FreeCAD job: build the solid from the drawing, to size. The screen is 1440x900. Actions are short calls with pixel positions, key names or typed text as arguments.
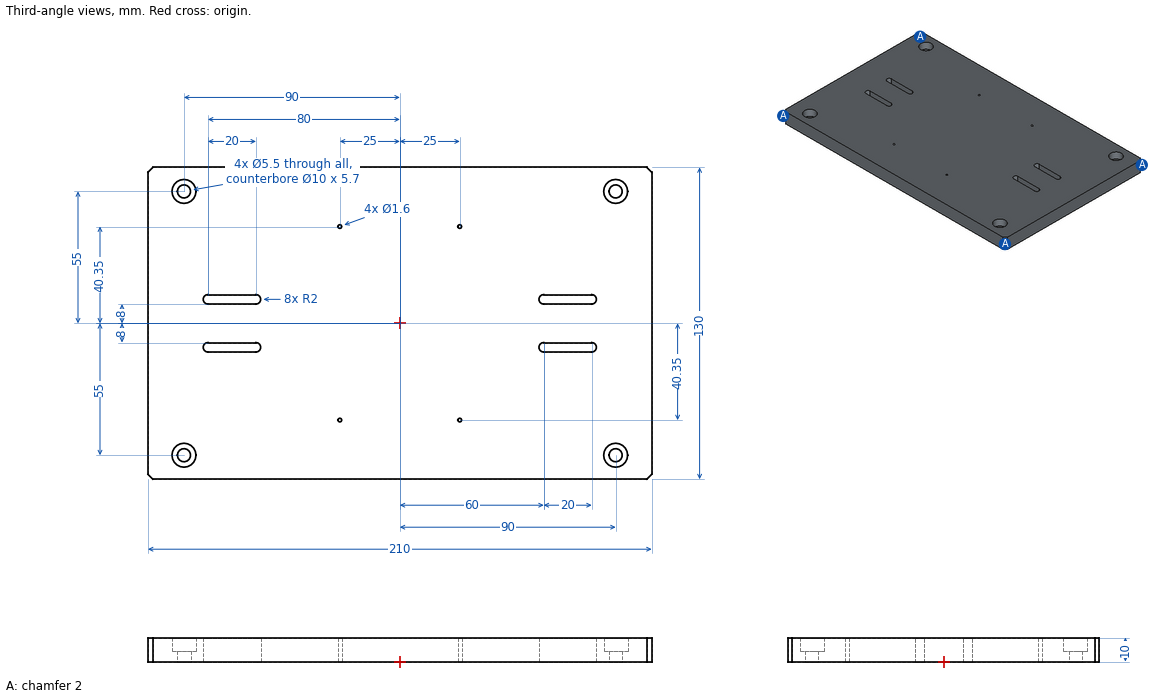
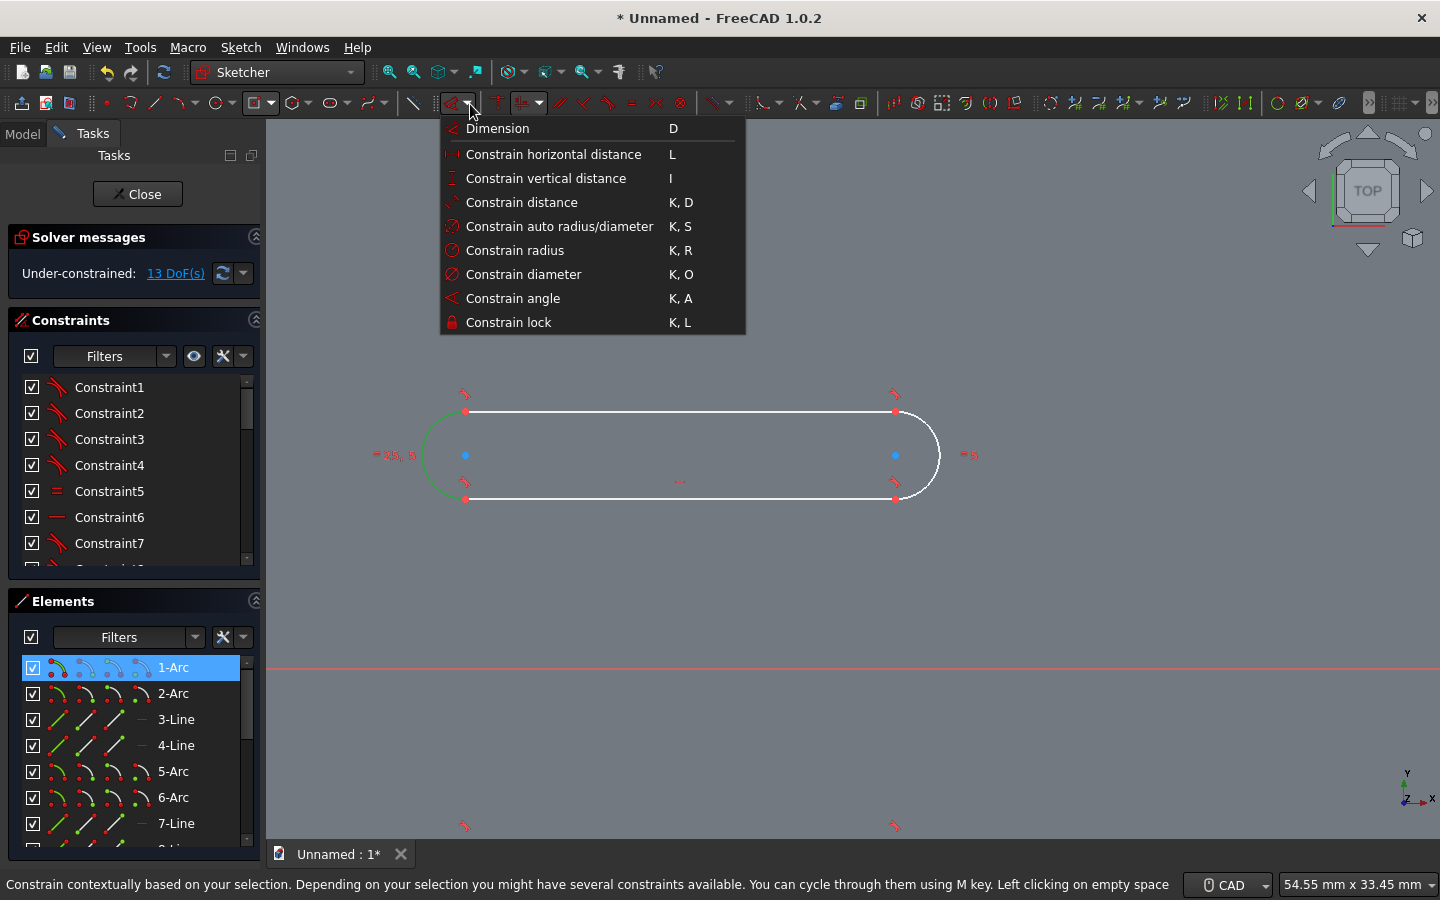
click(593, 250)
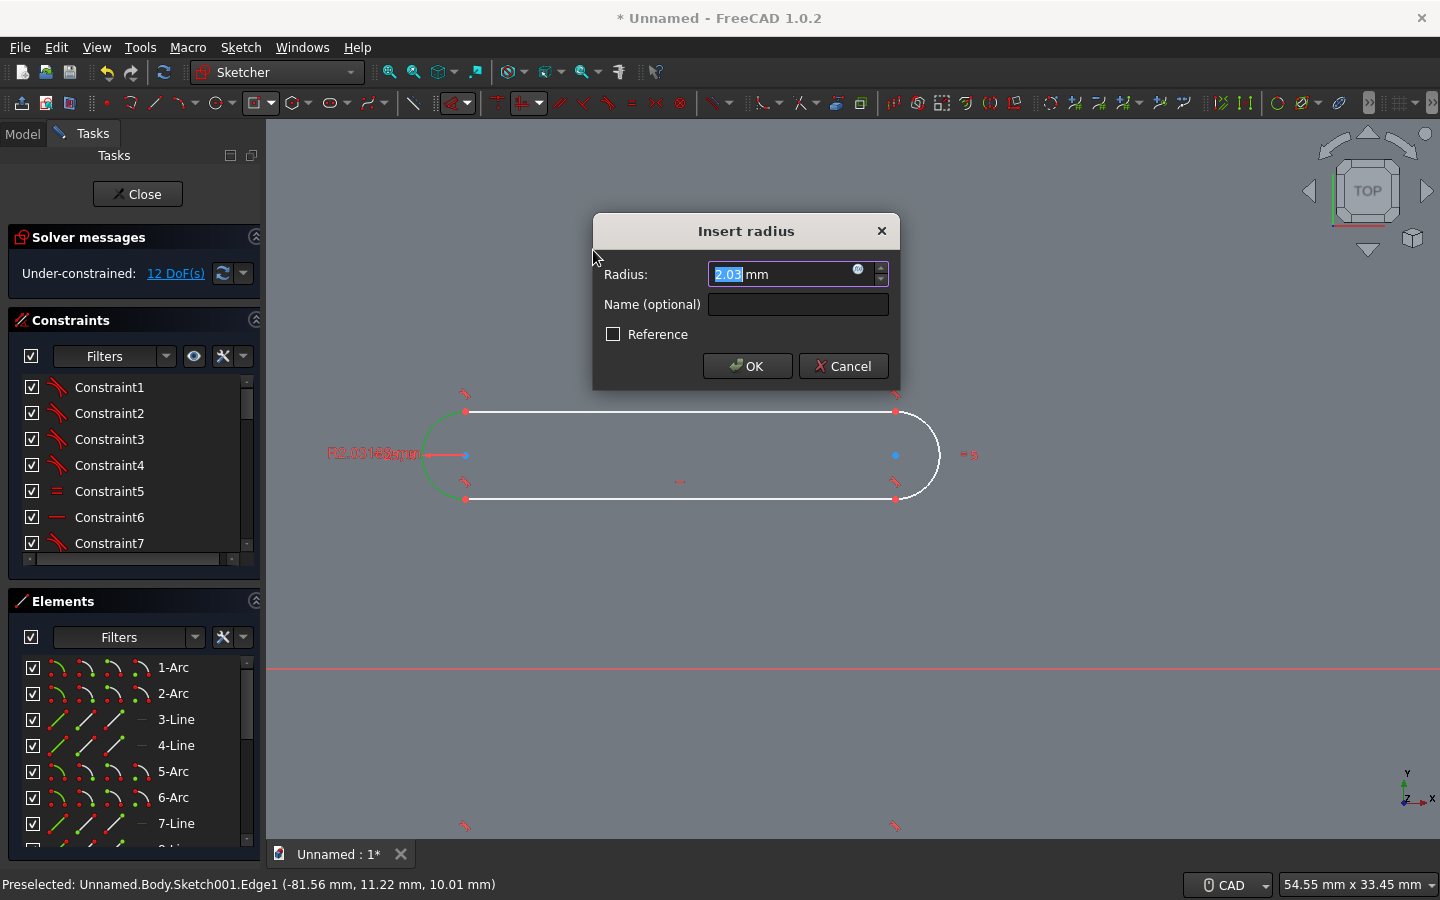
text(2)
key(Return)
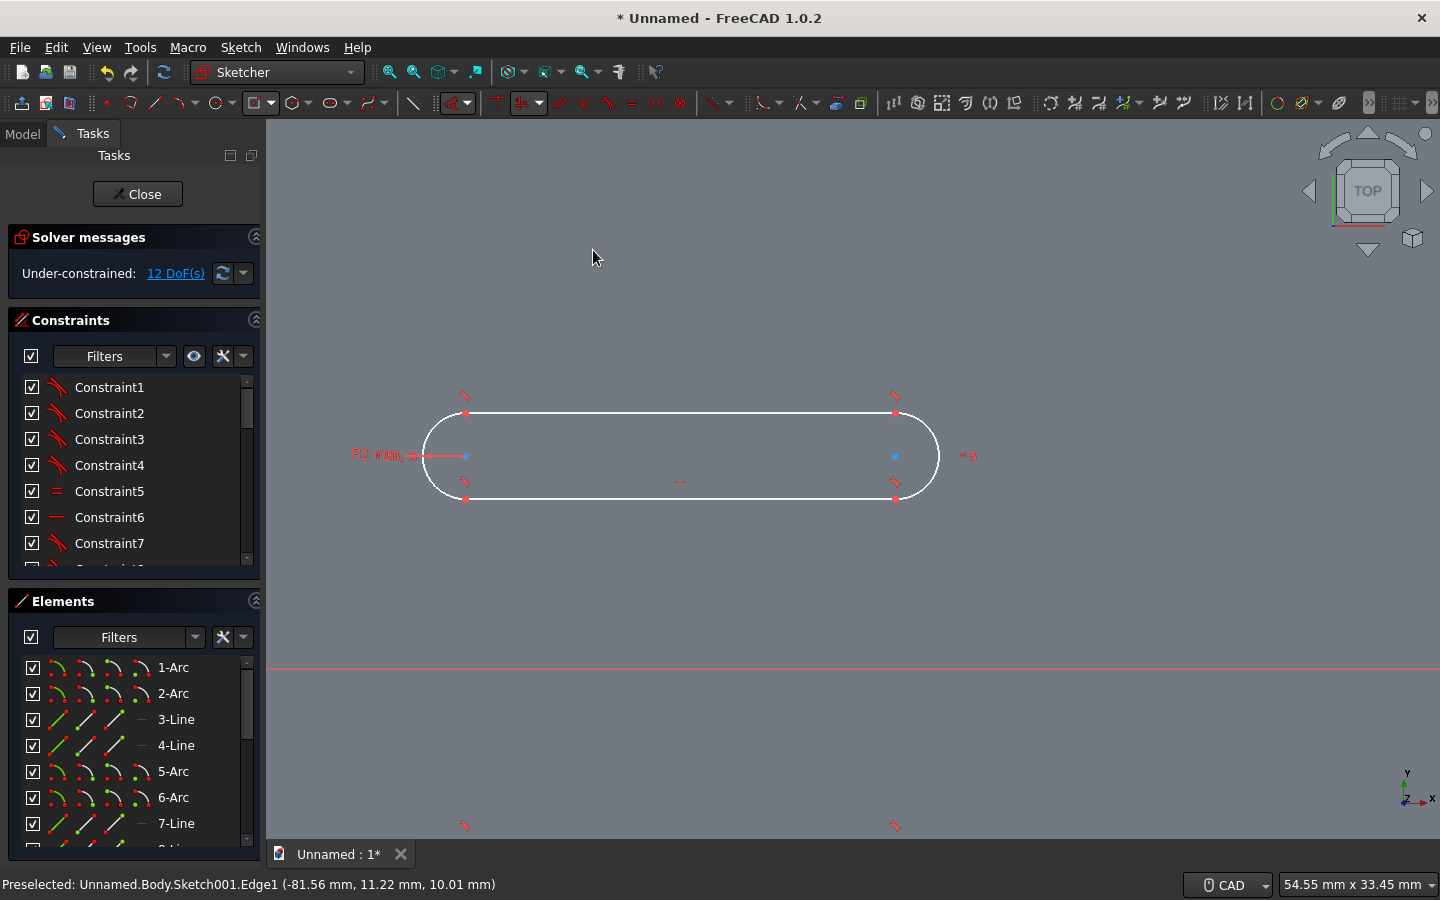
scroll(430, 431, down, 8)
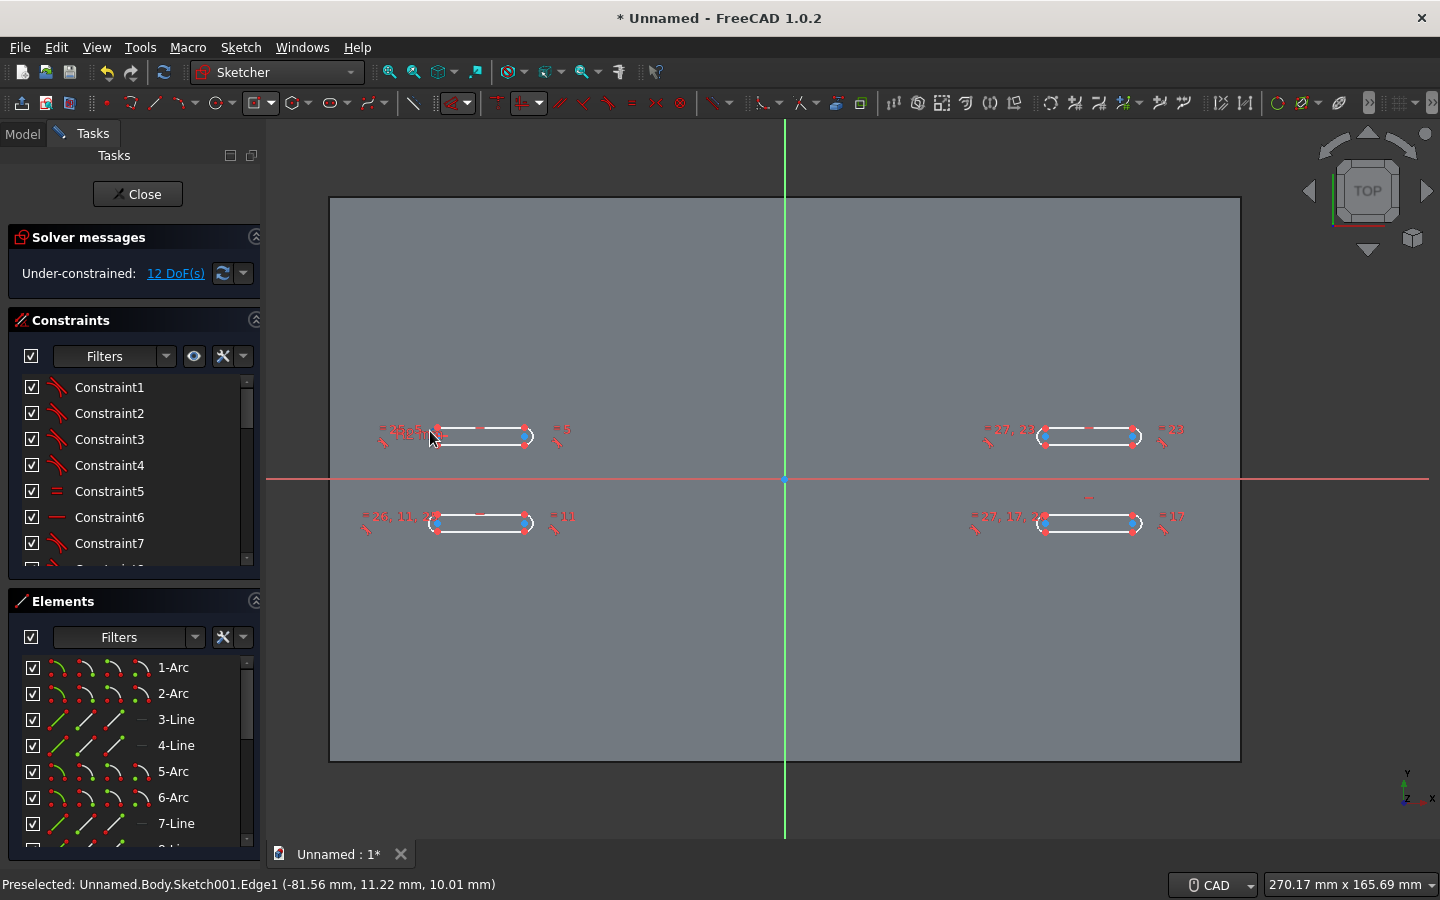
click(463, 428)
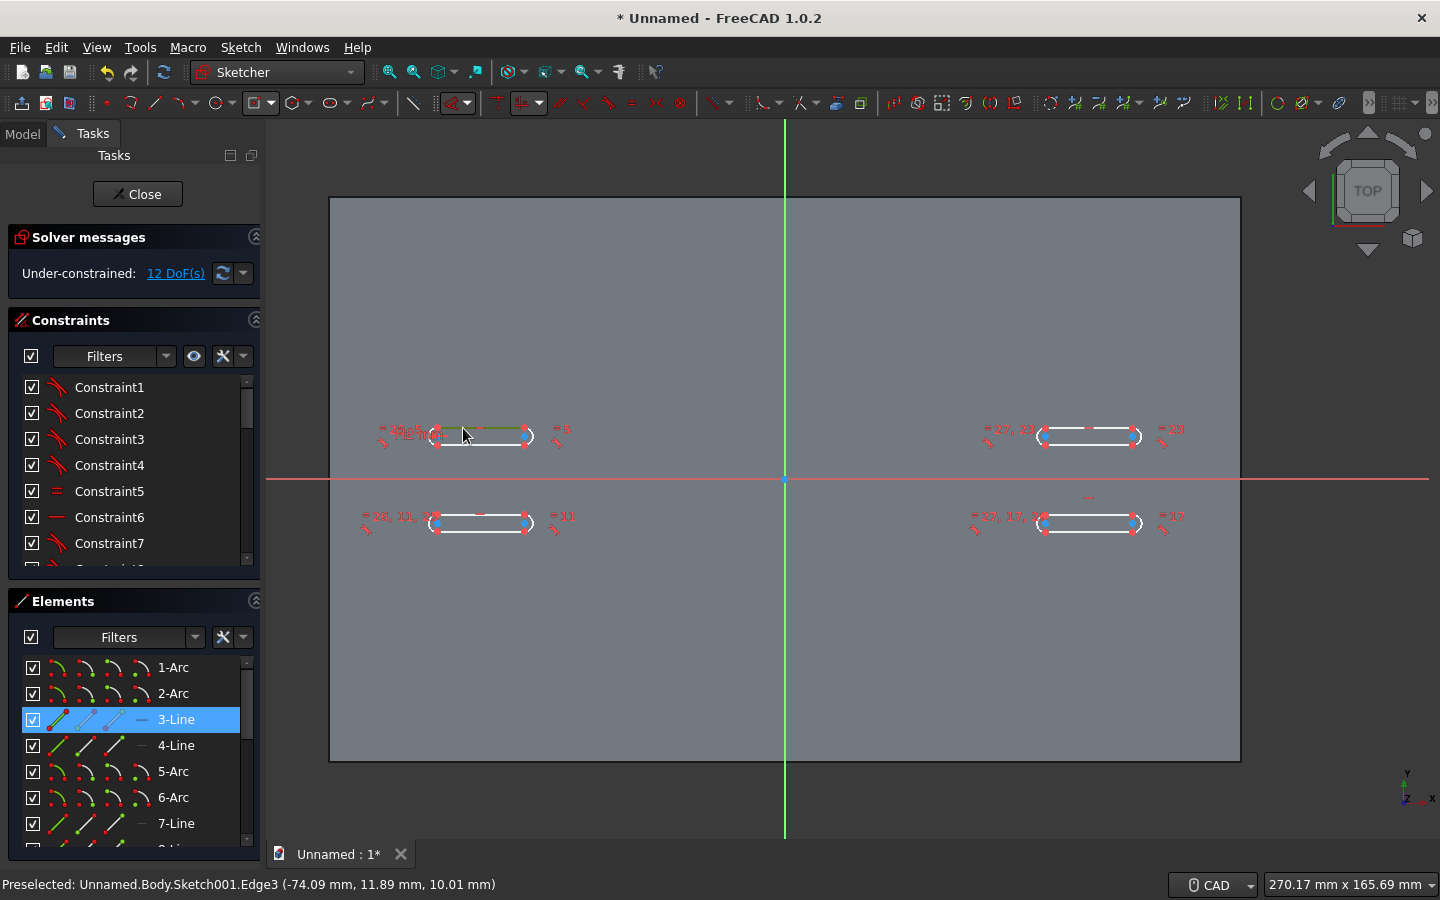
click(470, 104)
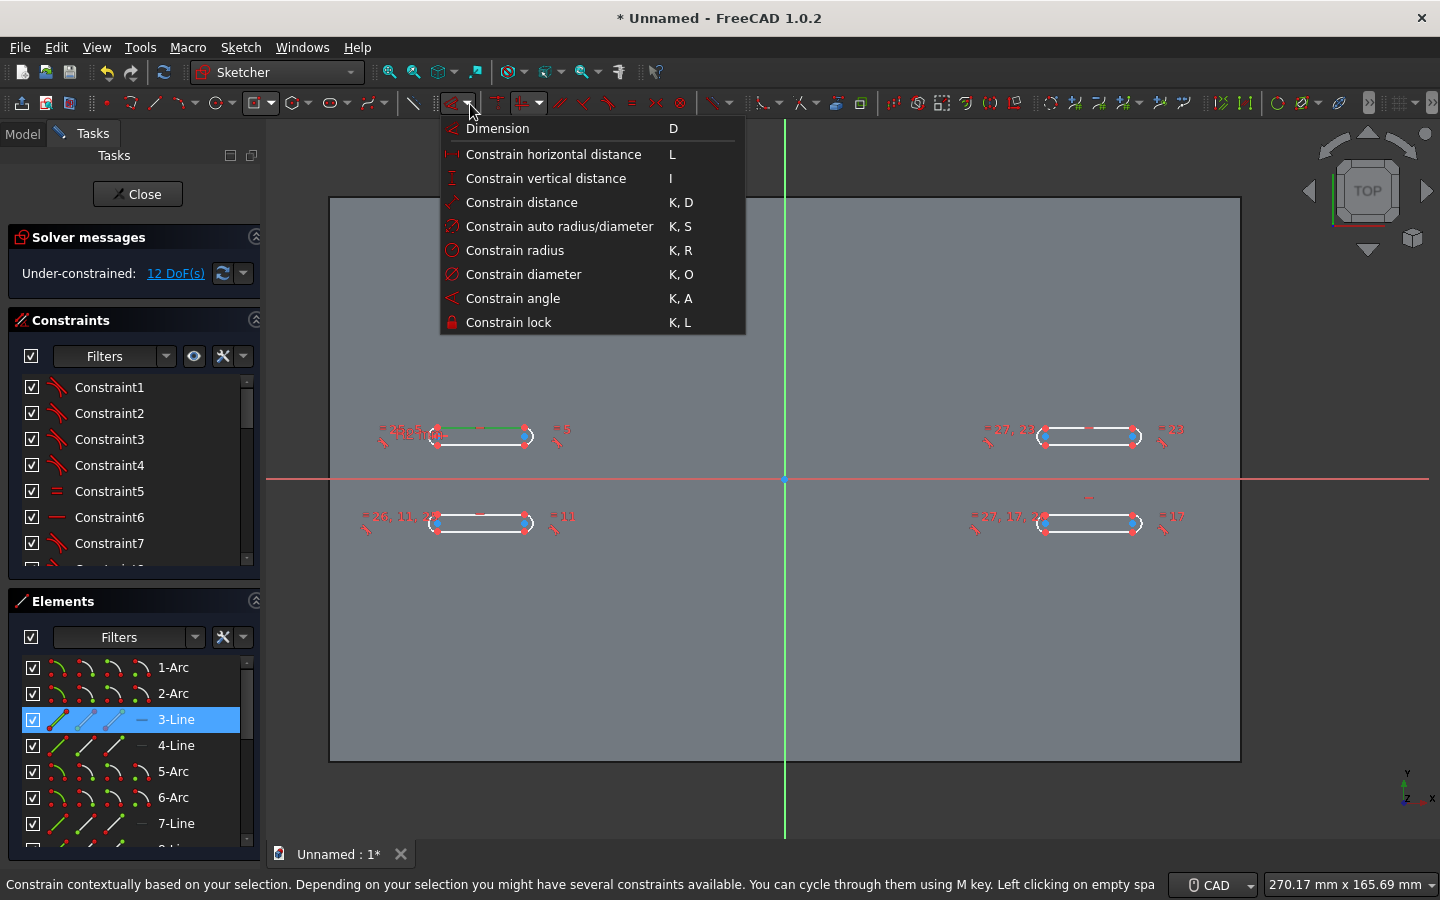
click(593, 154)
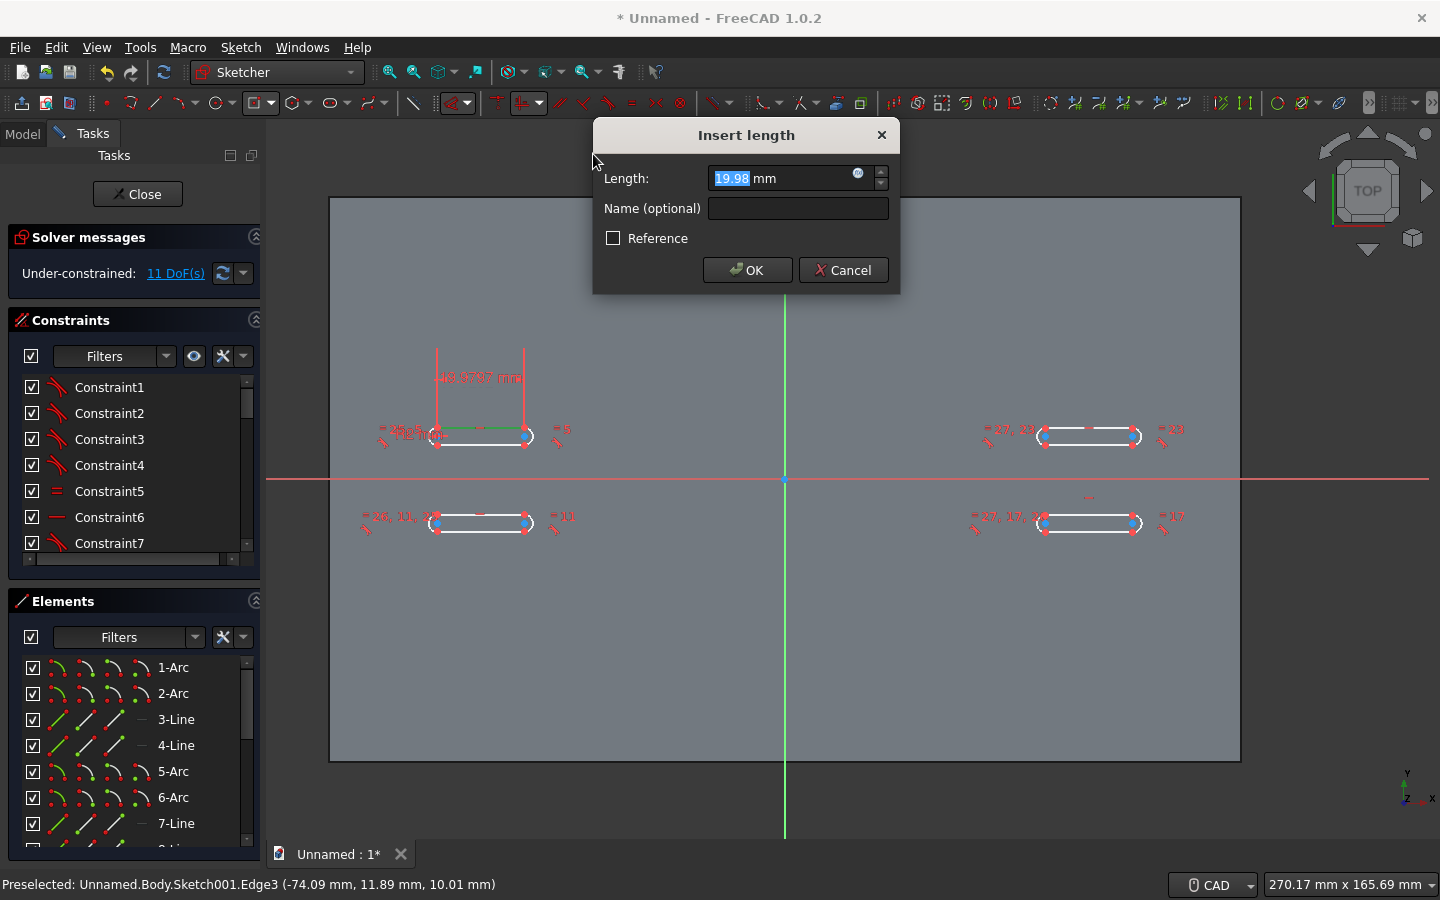
text(20)
key(Return)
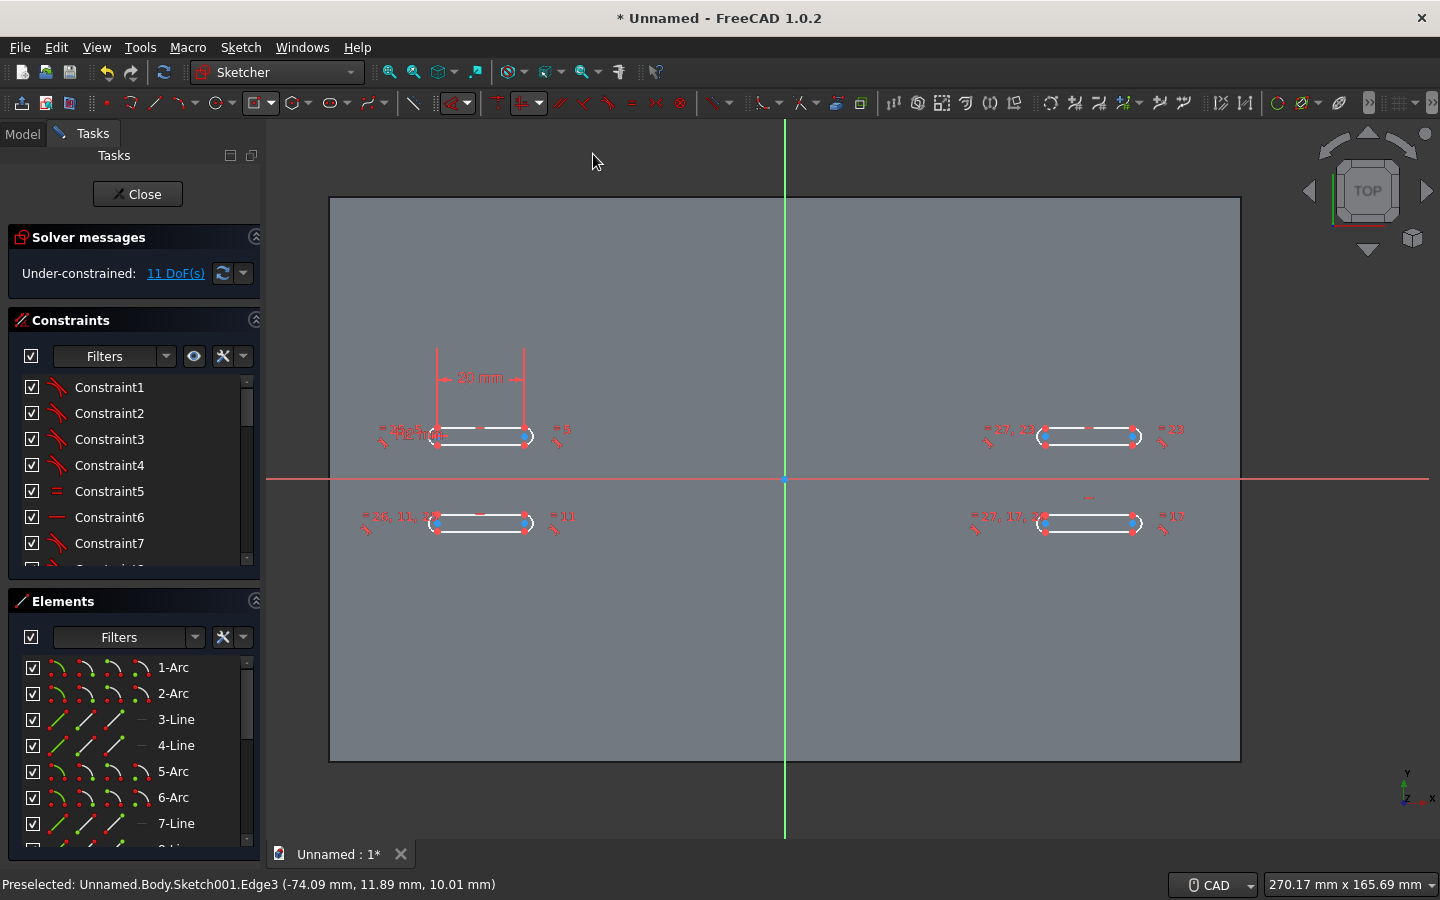
click(463, 515)